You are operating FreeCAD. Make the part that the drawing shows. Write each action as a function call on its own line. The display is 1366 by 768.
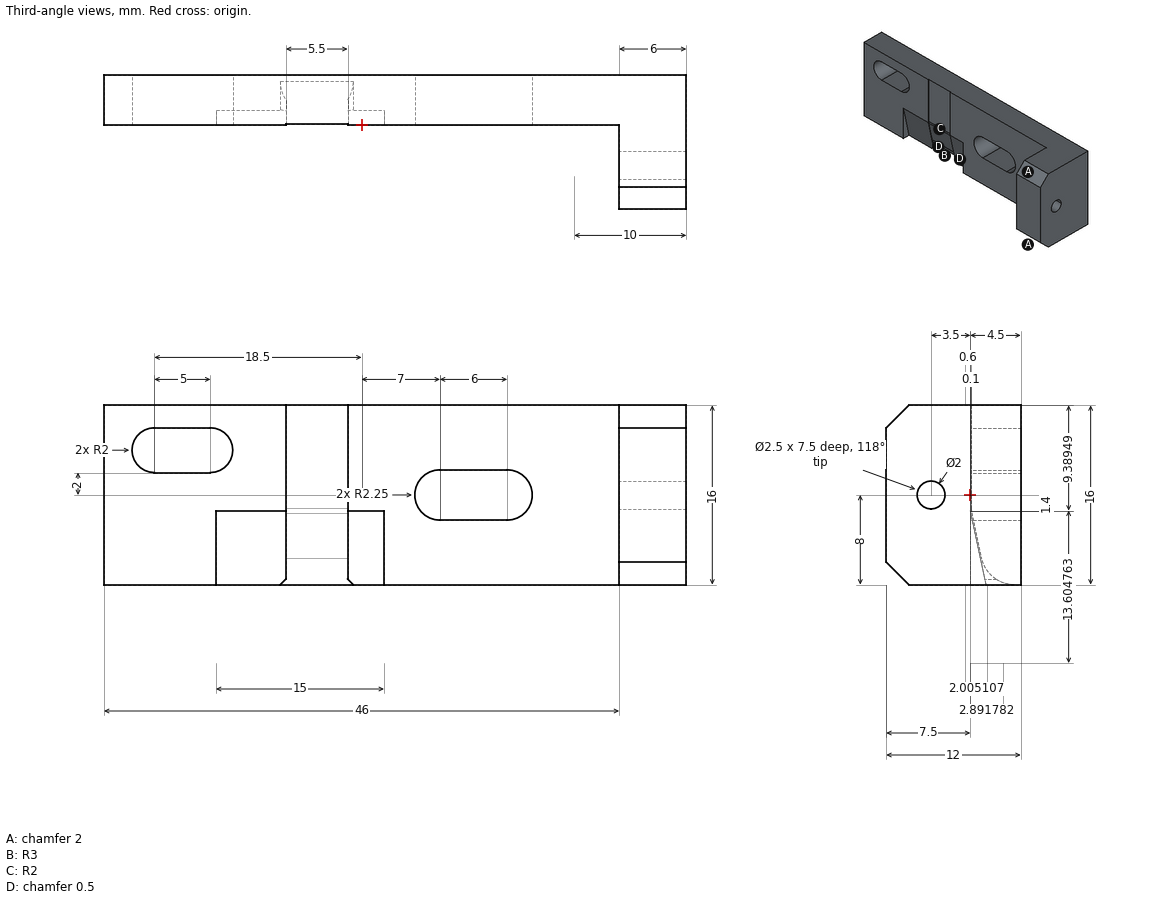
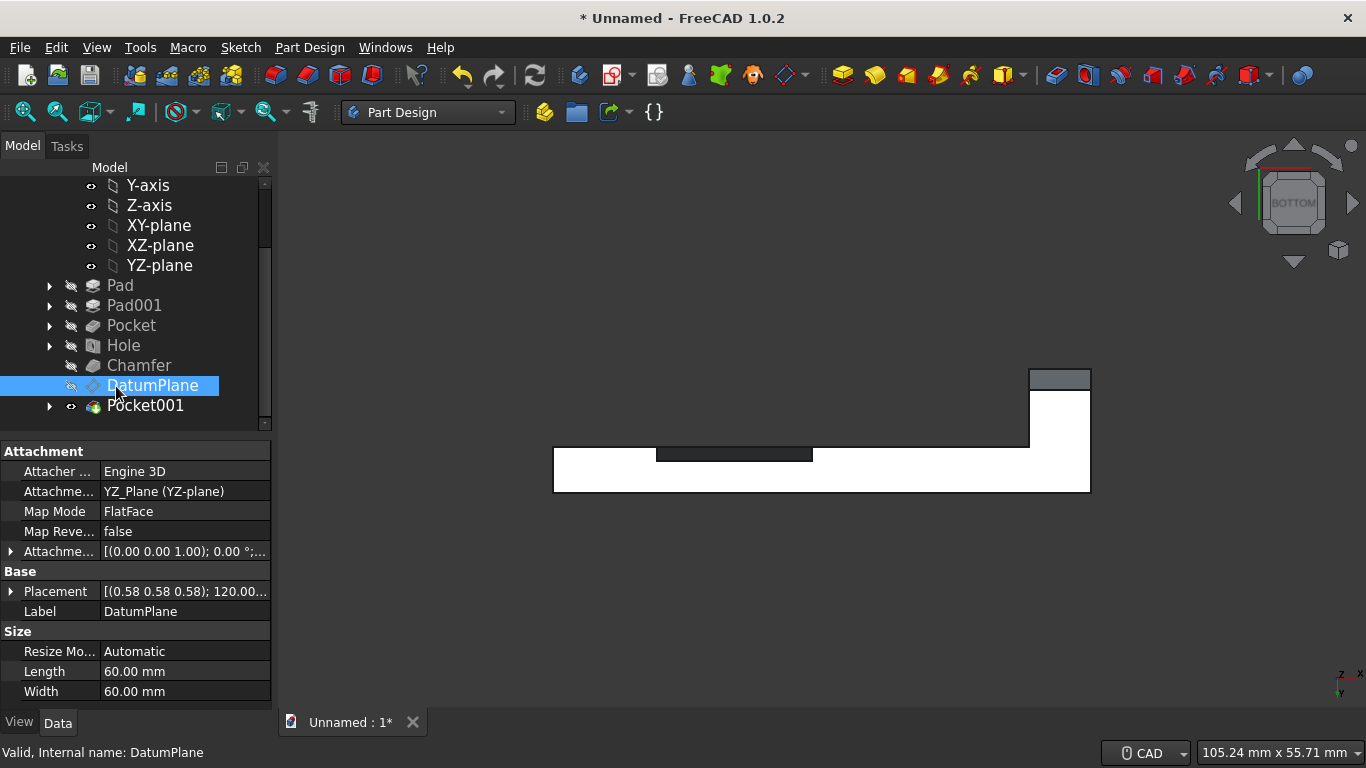
scroll(160, 301, down, 3)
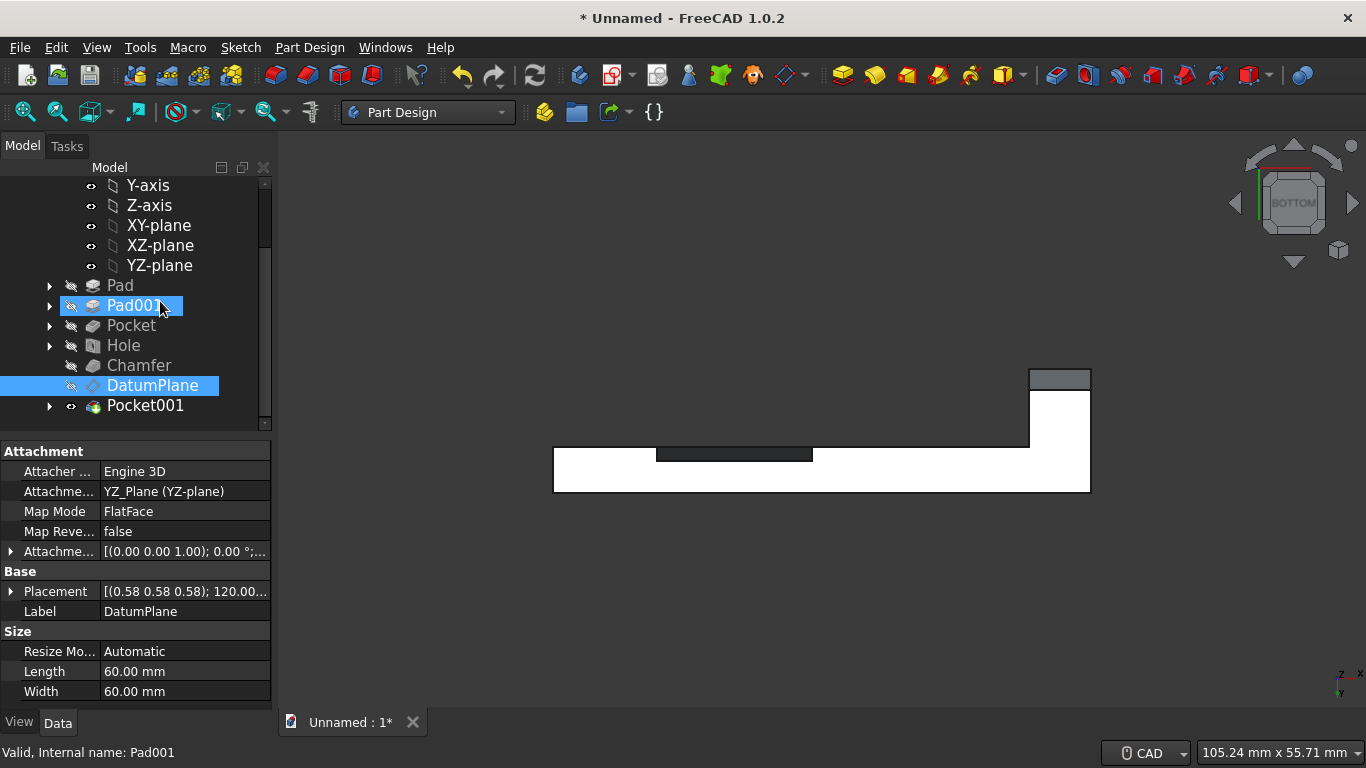
scroll(160, 301, up, 15)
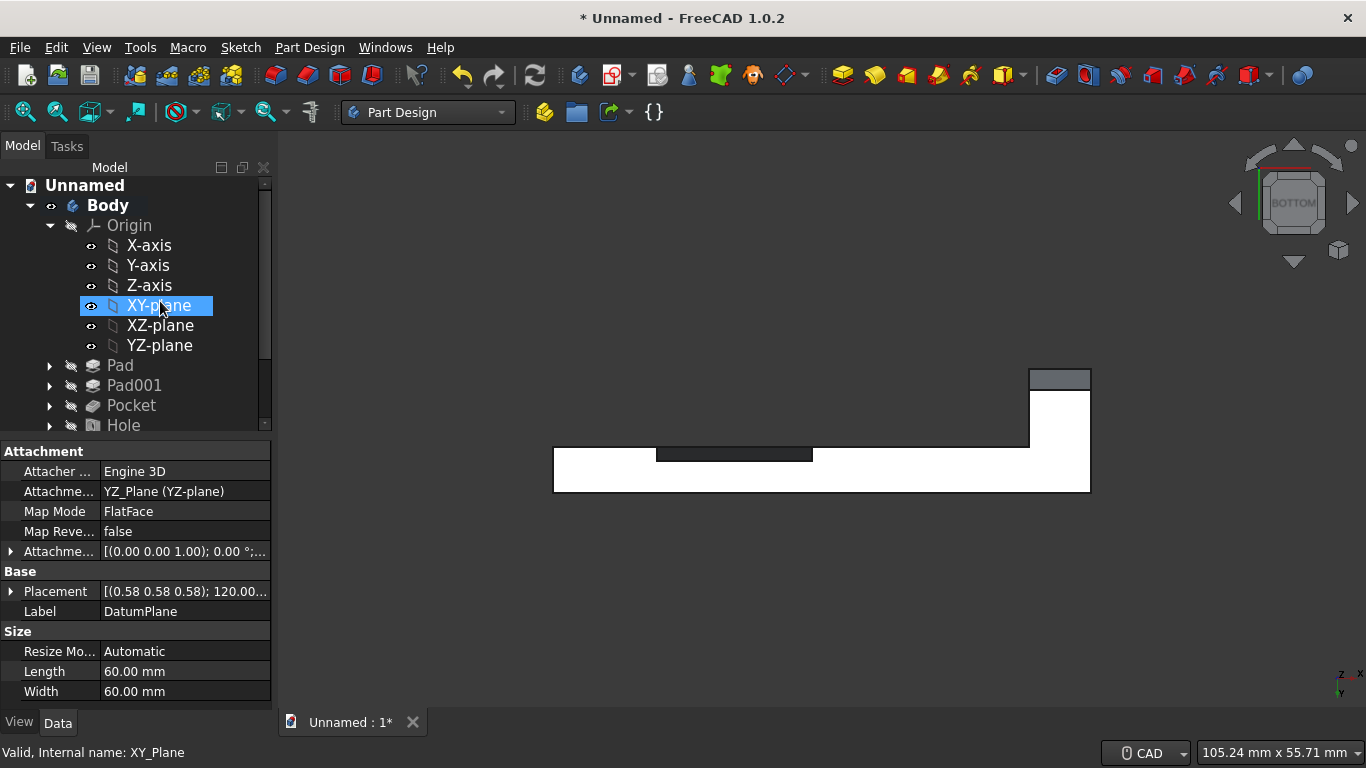
click(136, 346)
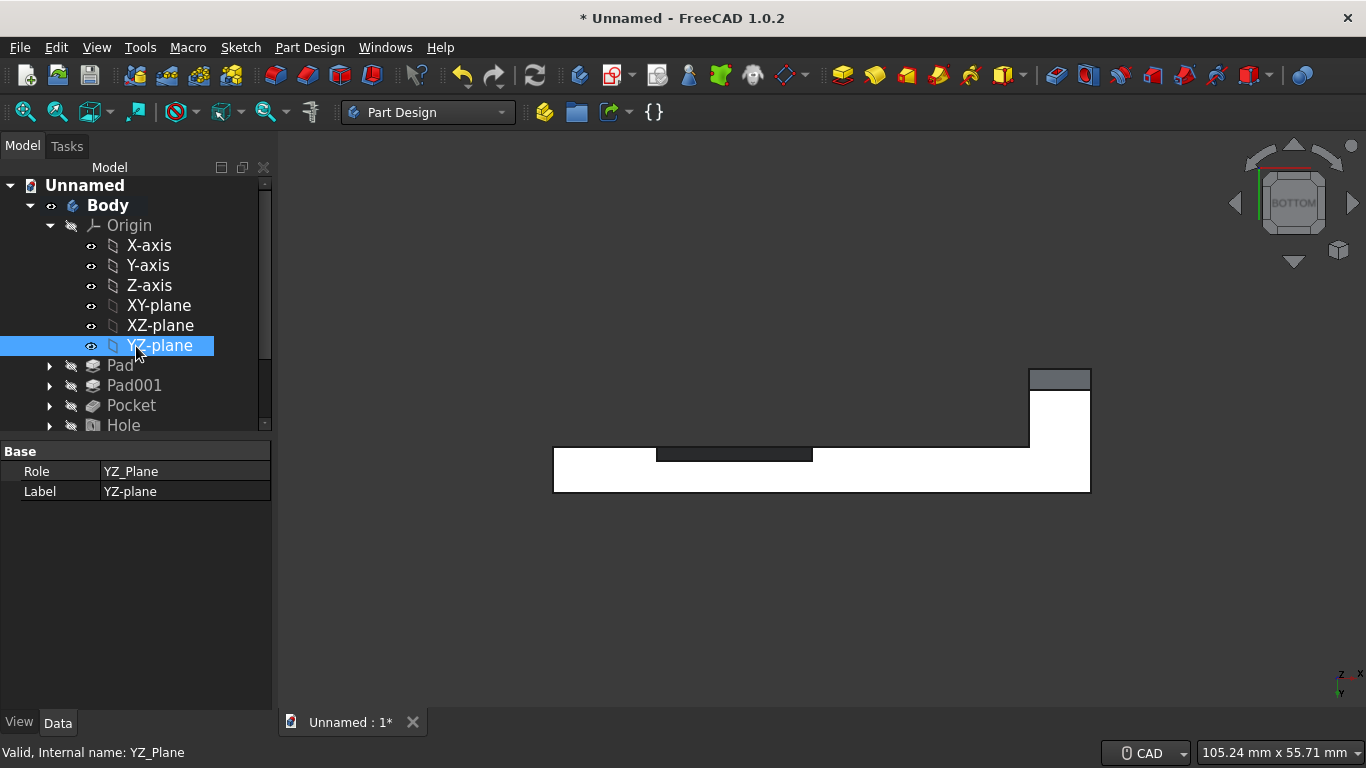
click(786, 76)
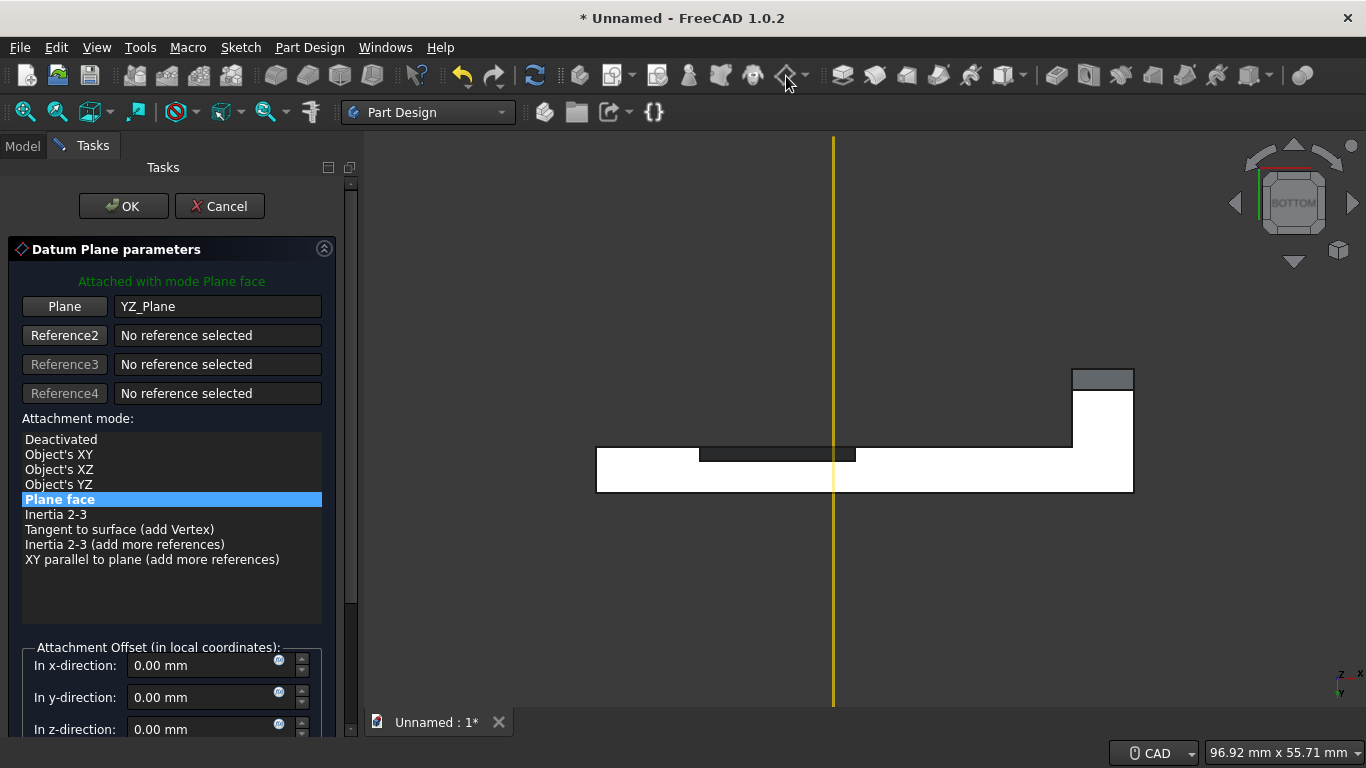
scroll(351, 456, down, 2)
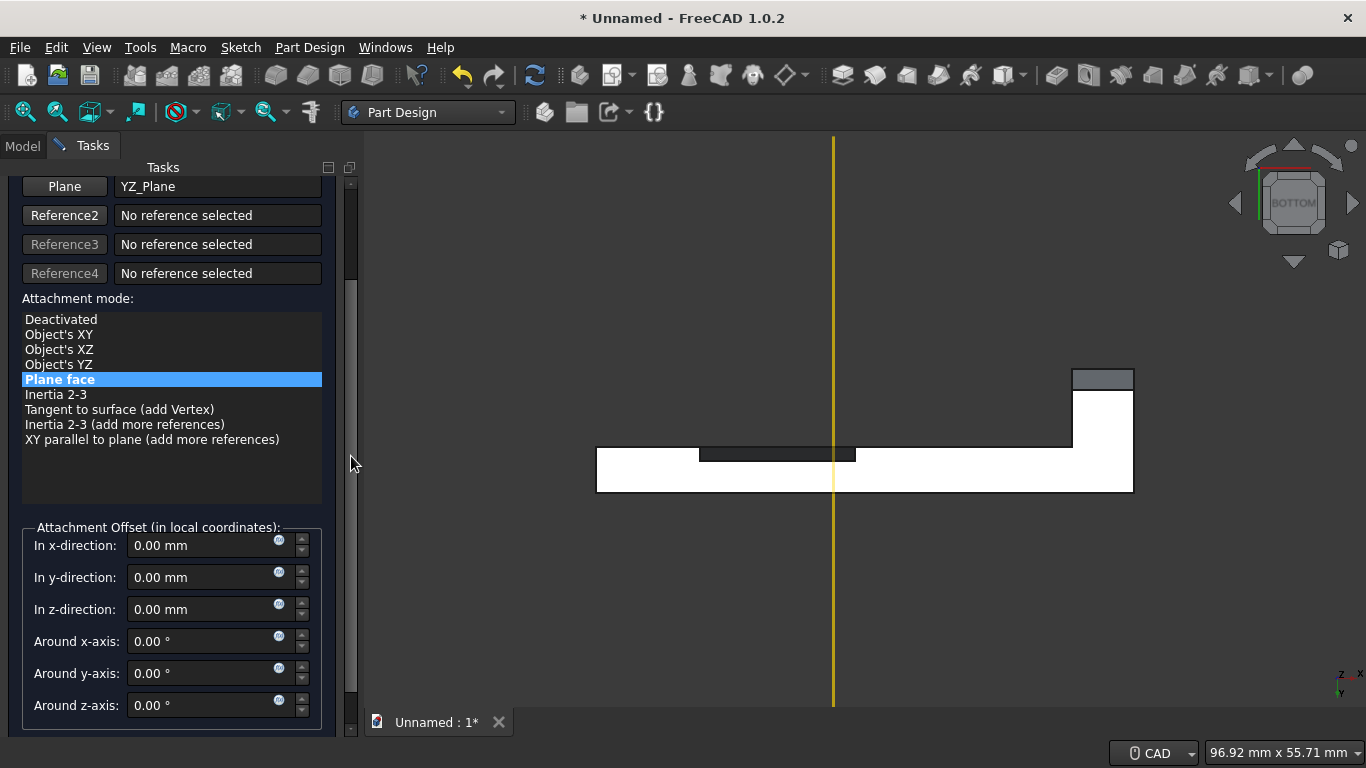
triple_click(210, 609)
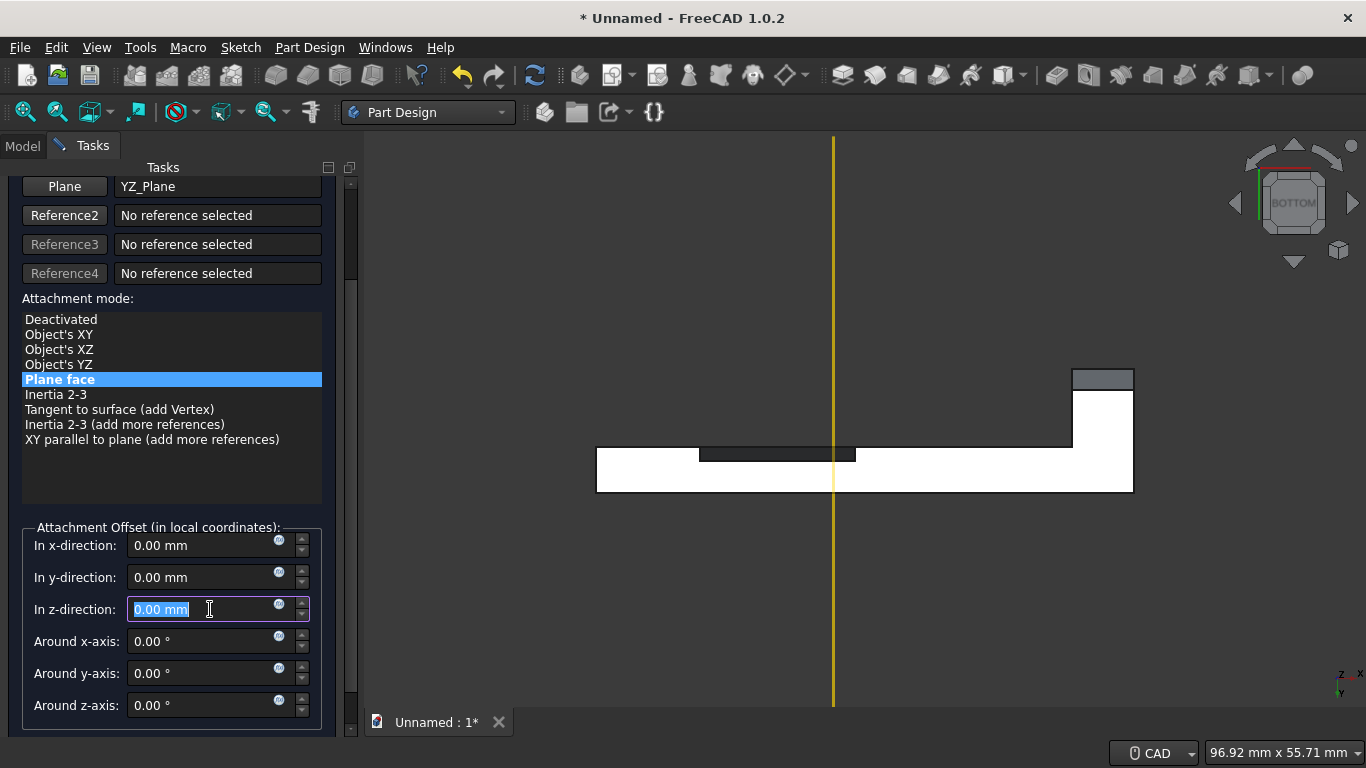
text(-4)
key(Tab)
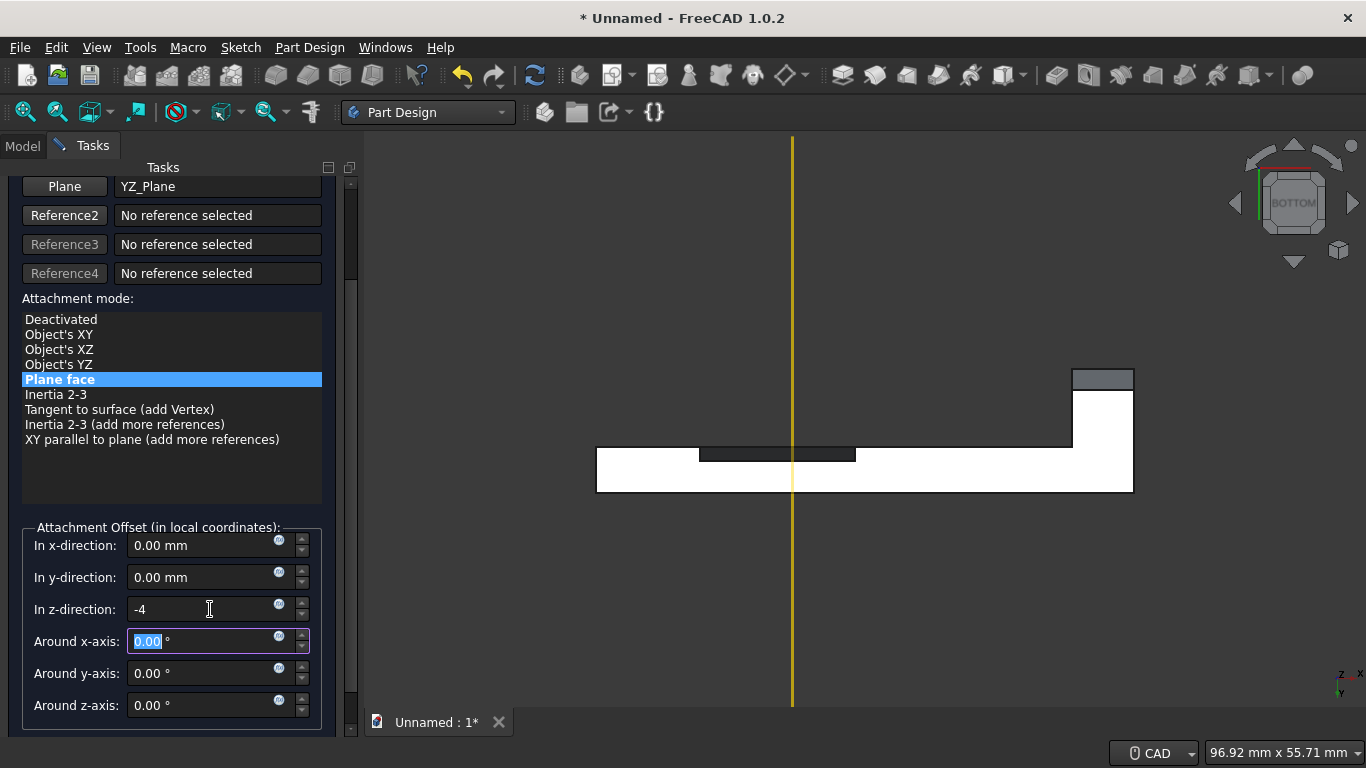
scroll(351, 456, up, 3)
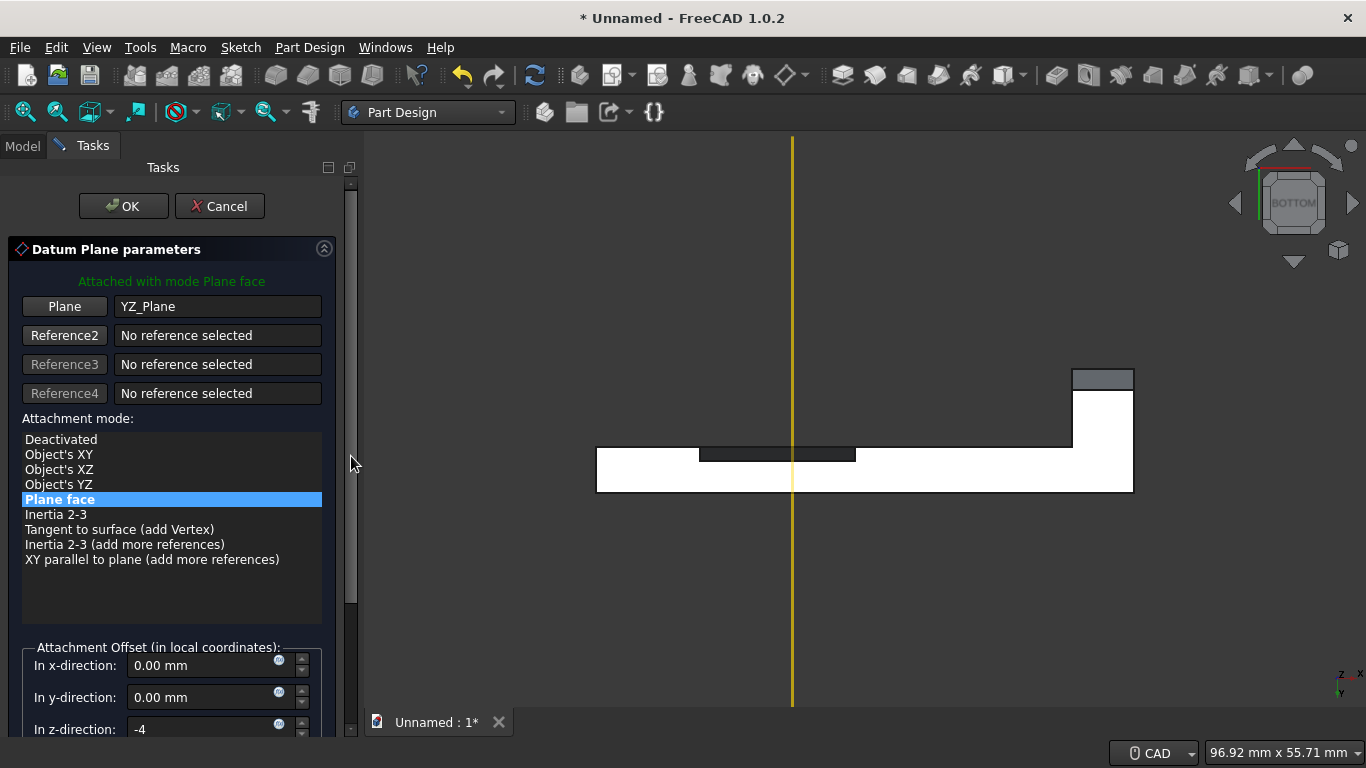
click(124, 206)